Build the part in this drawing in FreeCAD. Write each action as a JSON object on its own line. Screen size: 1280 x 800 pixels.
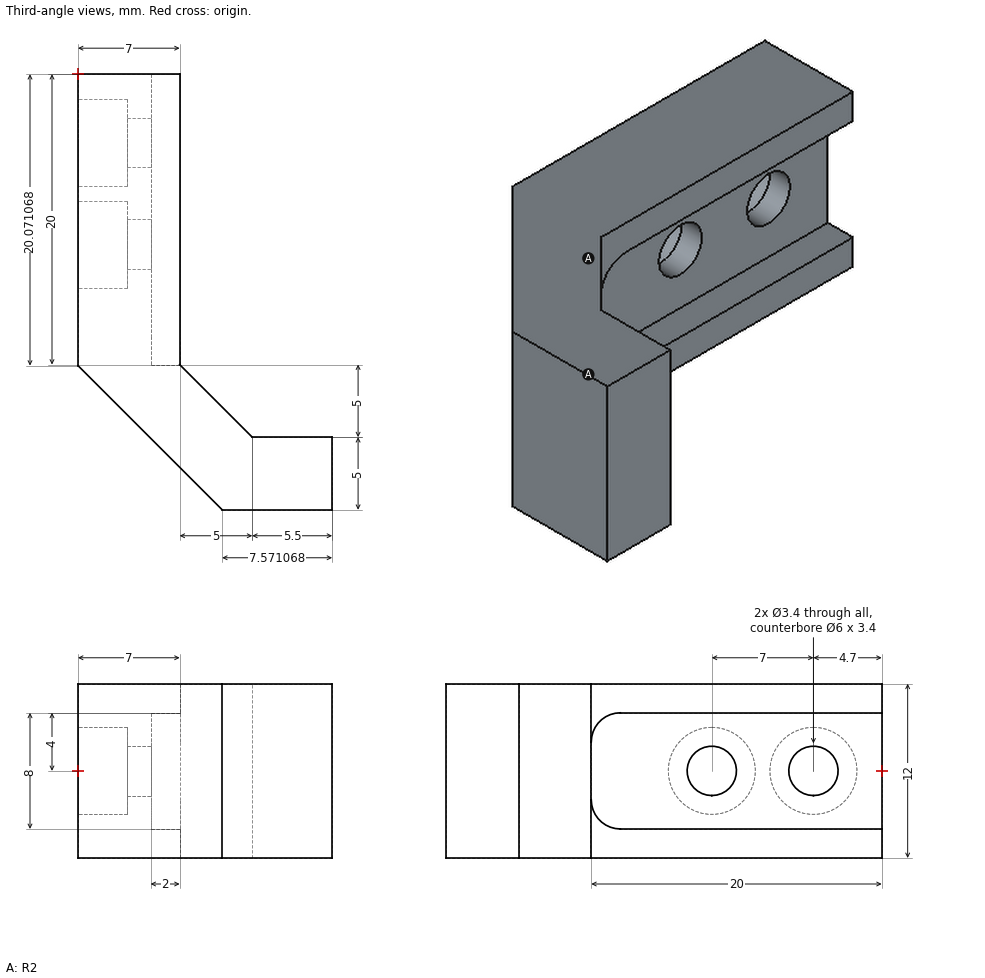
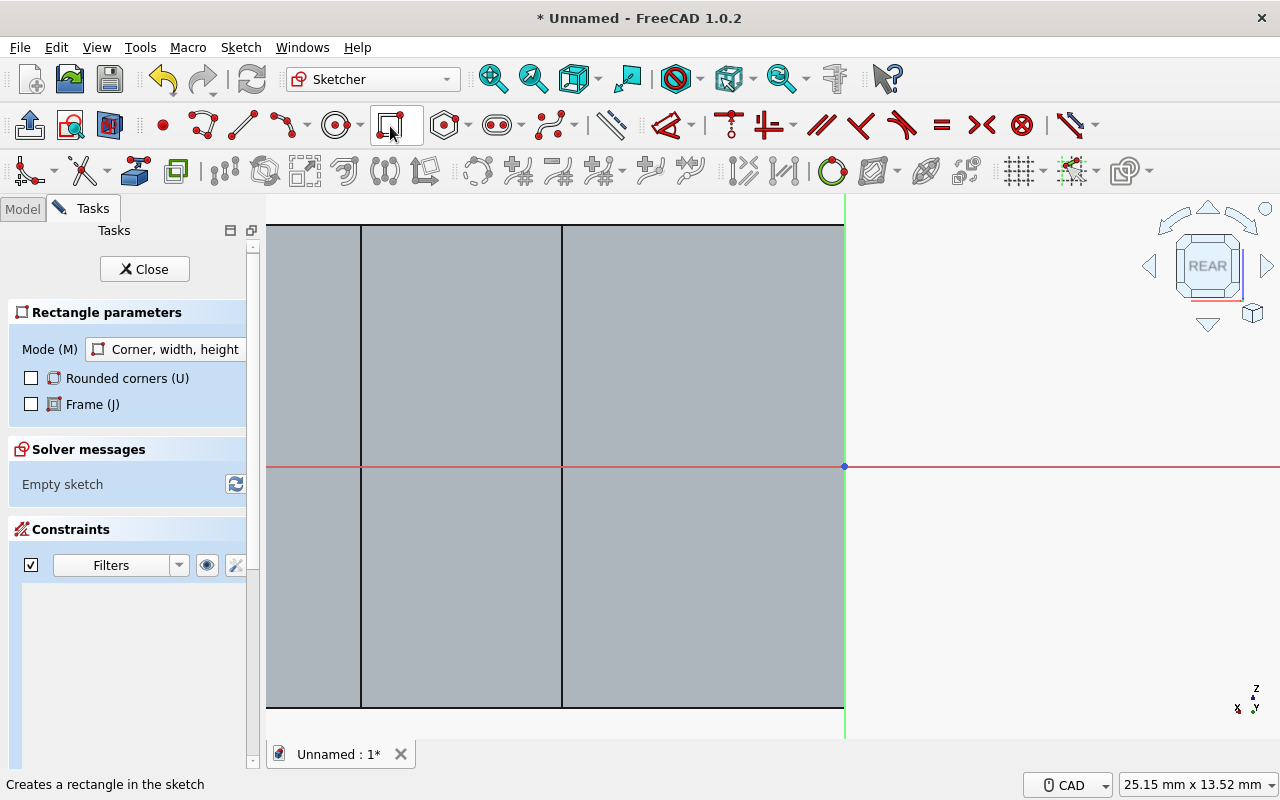
{"action": "left_click", "coordinate": [562, 305]}
{"action": "left_click", "coordinate": [643, 628]}
{"action": "key", "text": "Escape"}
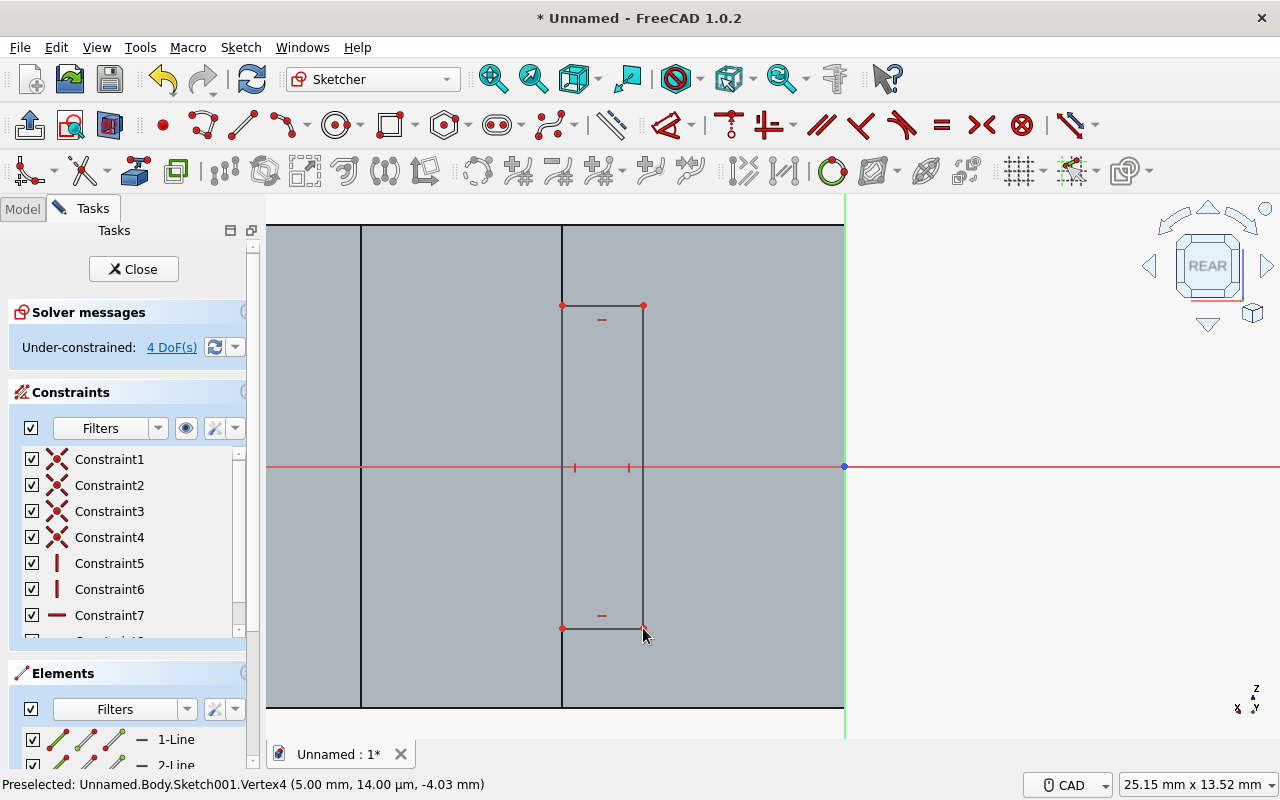
{"action": "left_click", "coordinate": [666, 126]}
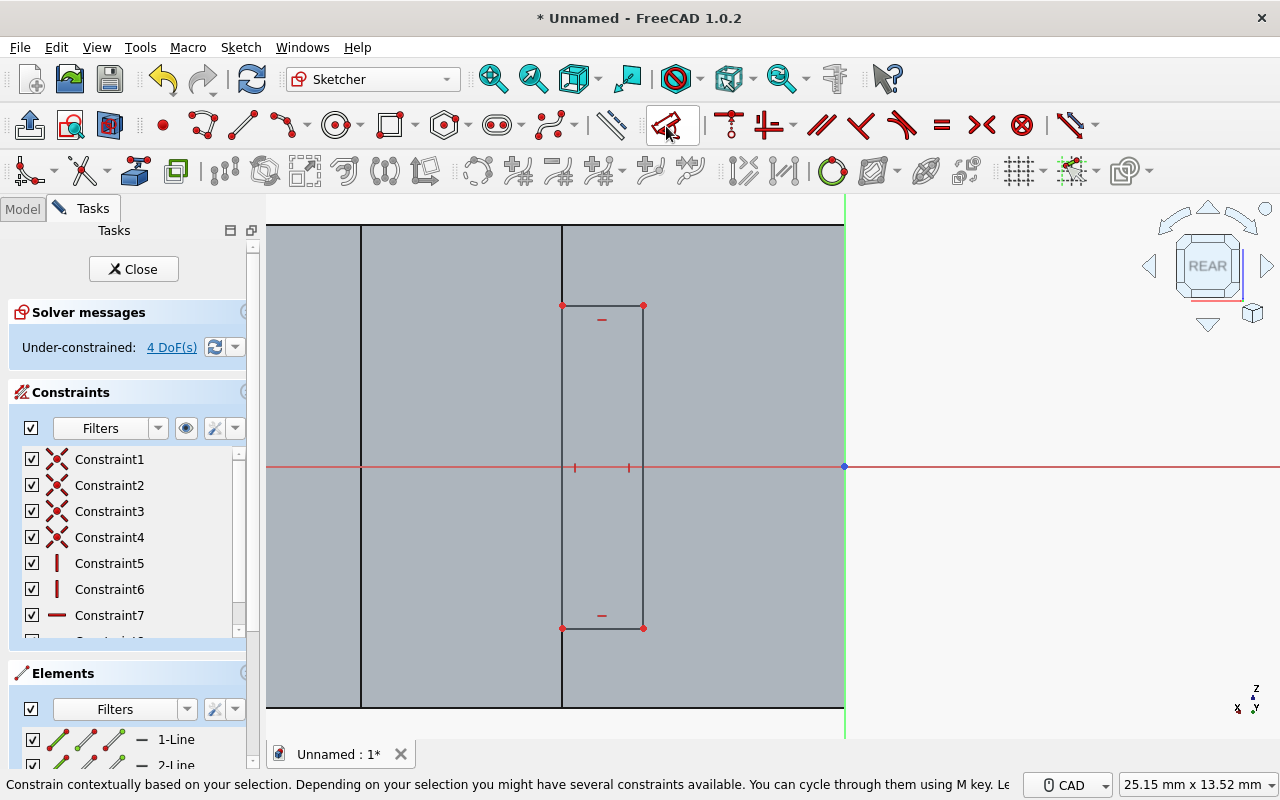
{"action": "left_click", "coordinate": [562, 403]}
{"action": "left_click", "coordinate": [528, 393]}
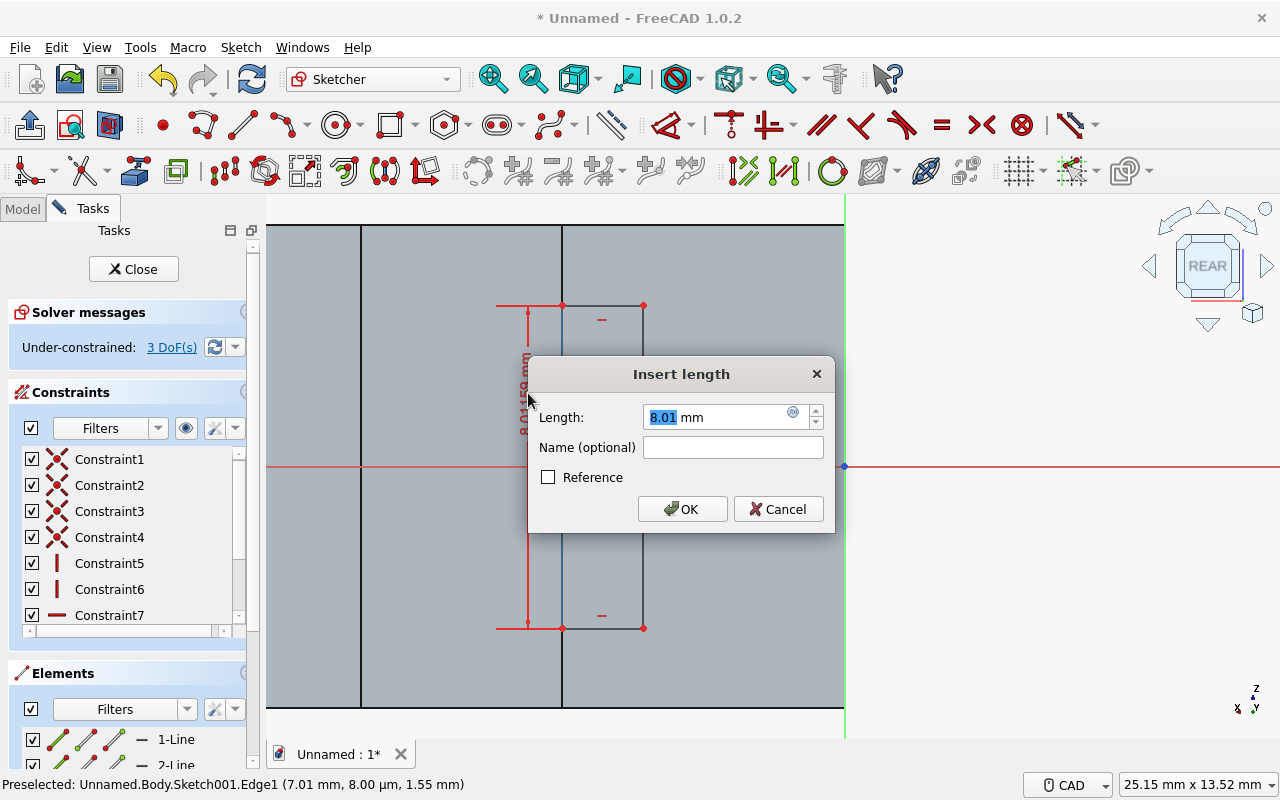
{"action": "type", "text": "8"}
{"action": "key", "text": "Return"}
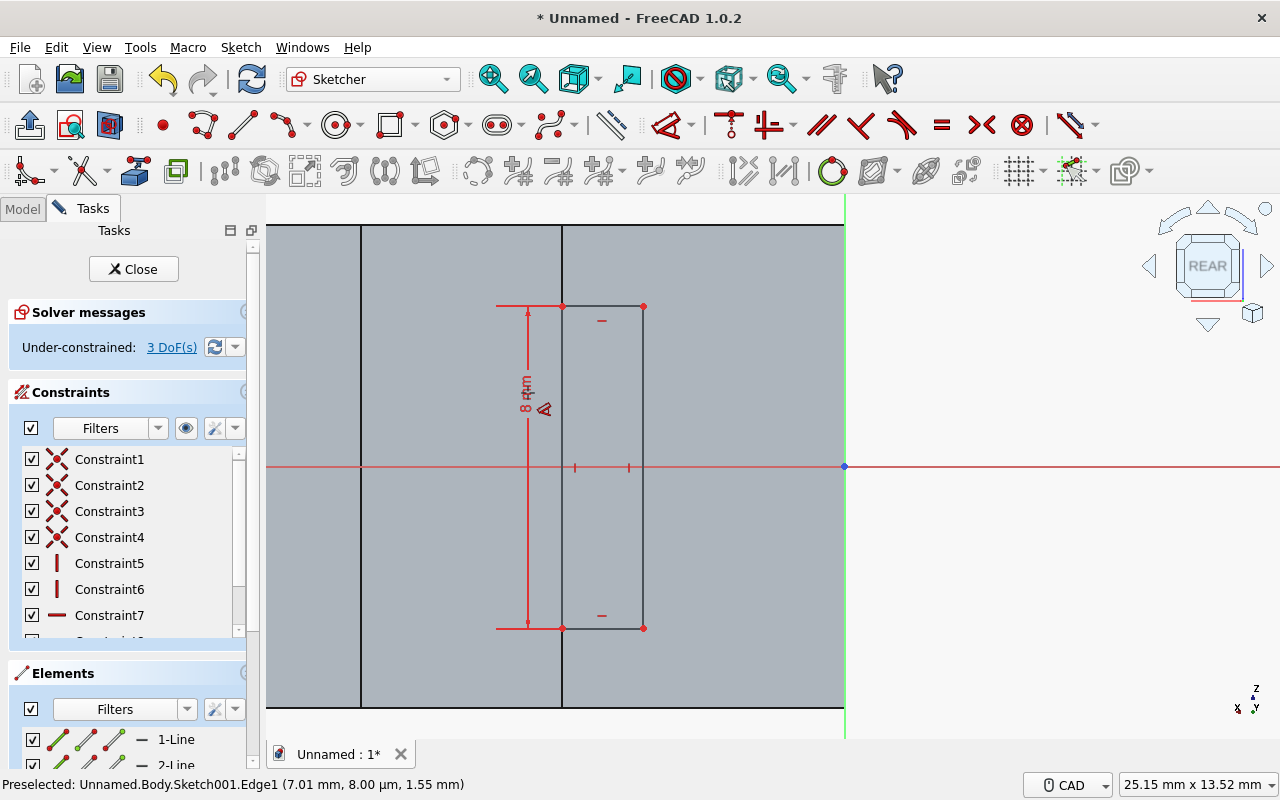
{"action": "left_click", "coordinate": [586, 629]}
{"action": "left_click", "coordinate": [602, 663]}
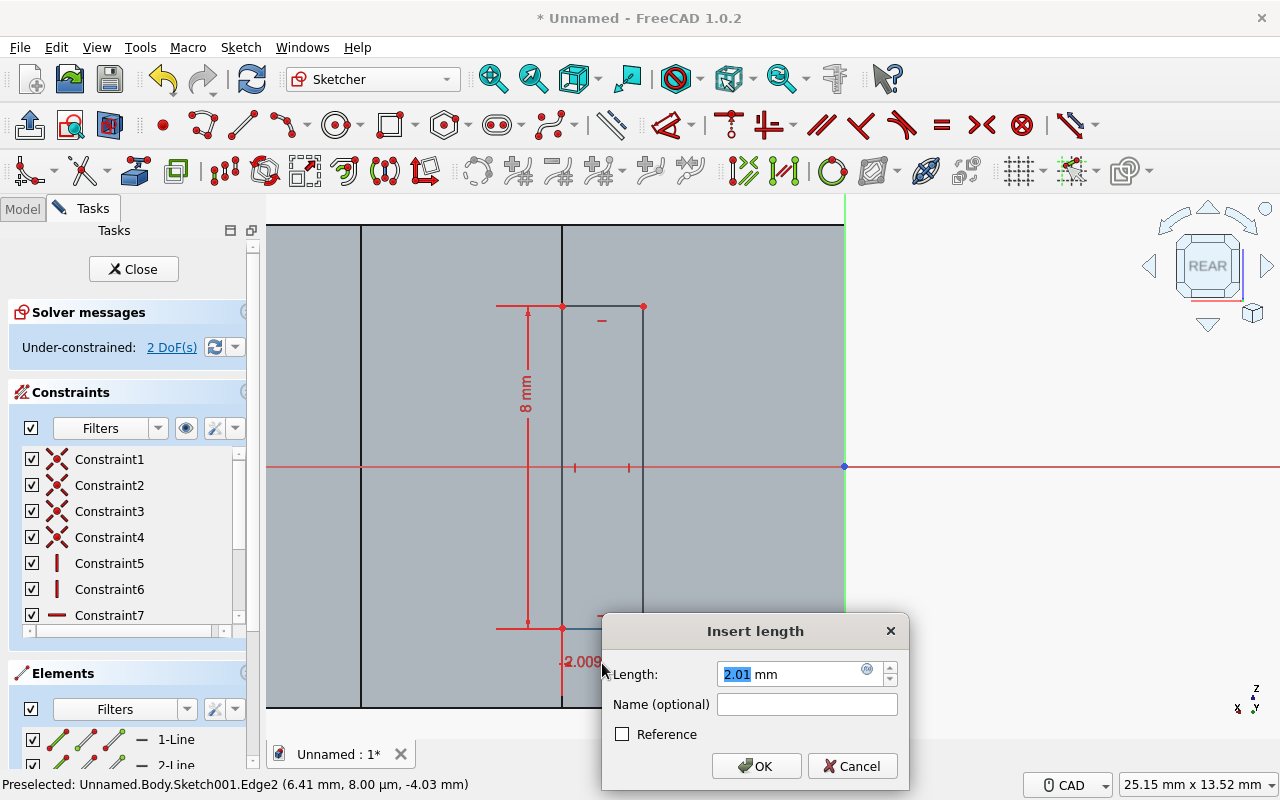
{"action": "type", "text": "2"}
{"action": "key", "text": "Return"}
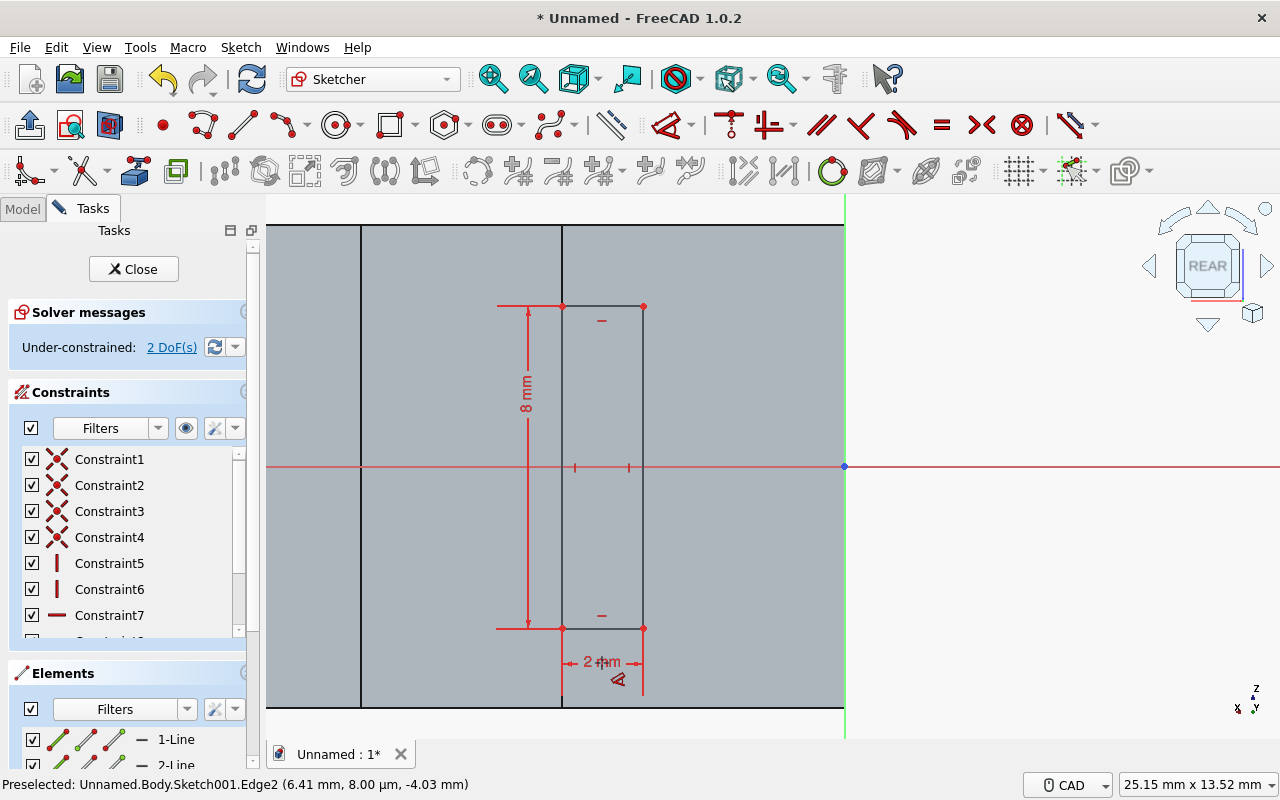
{"action": "left_click", "coordinate": [562, 306]}
{"action": "left_click", "coordinate": [703, 272]}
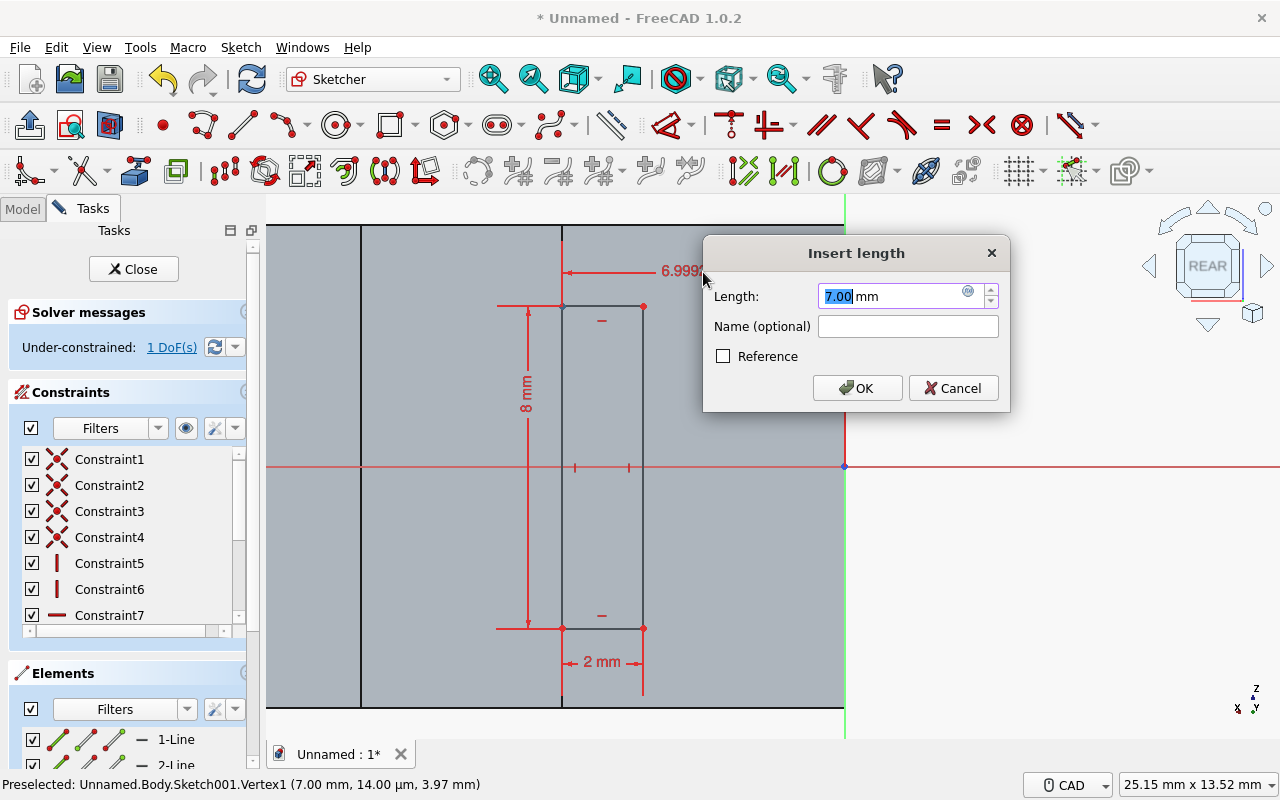
{"action": "type", "text": "7"}
{"action": "key", "text": "Return"}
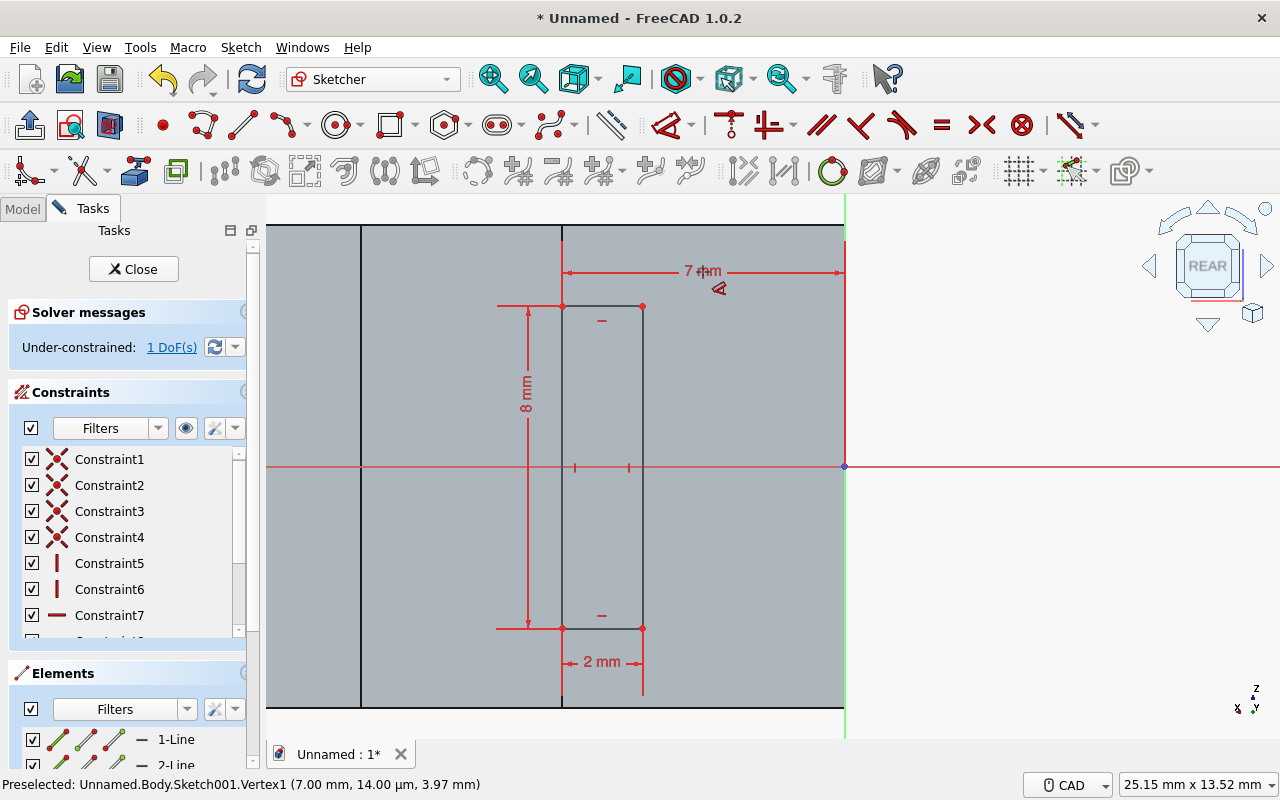
{"action": "left_click", "coordinate": [562, 306]}
{"action": "left_click", "coordinate": [879, 386]}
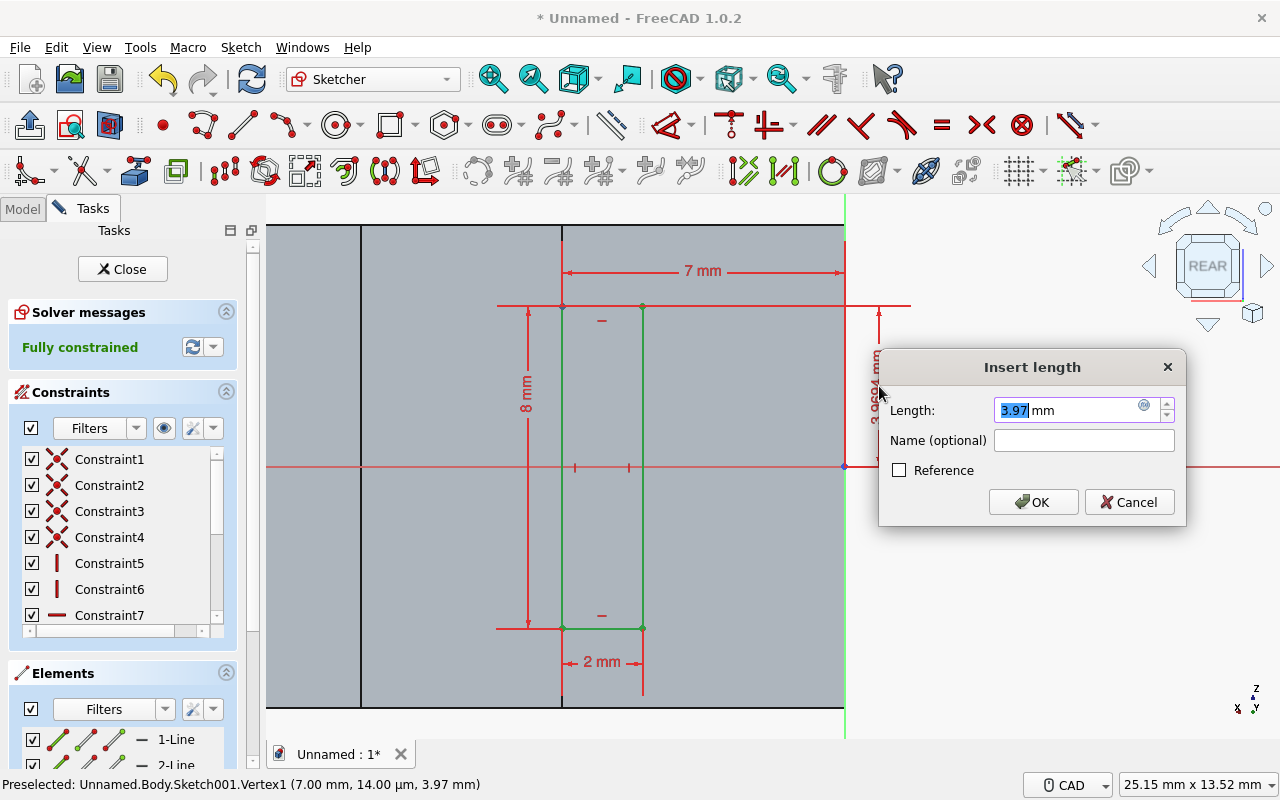
{"action": "type", "text": "4"}
{"action": "key", "text": "Return"}
{"action": "key", "text": "Escape"}